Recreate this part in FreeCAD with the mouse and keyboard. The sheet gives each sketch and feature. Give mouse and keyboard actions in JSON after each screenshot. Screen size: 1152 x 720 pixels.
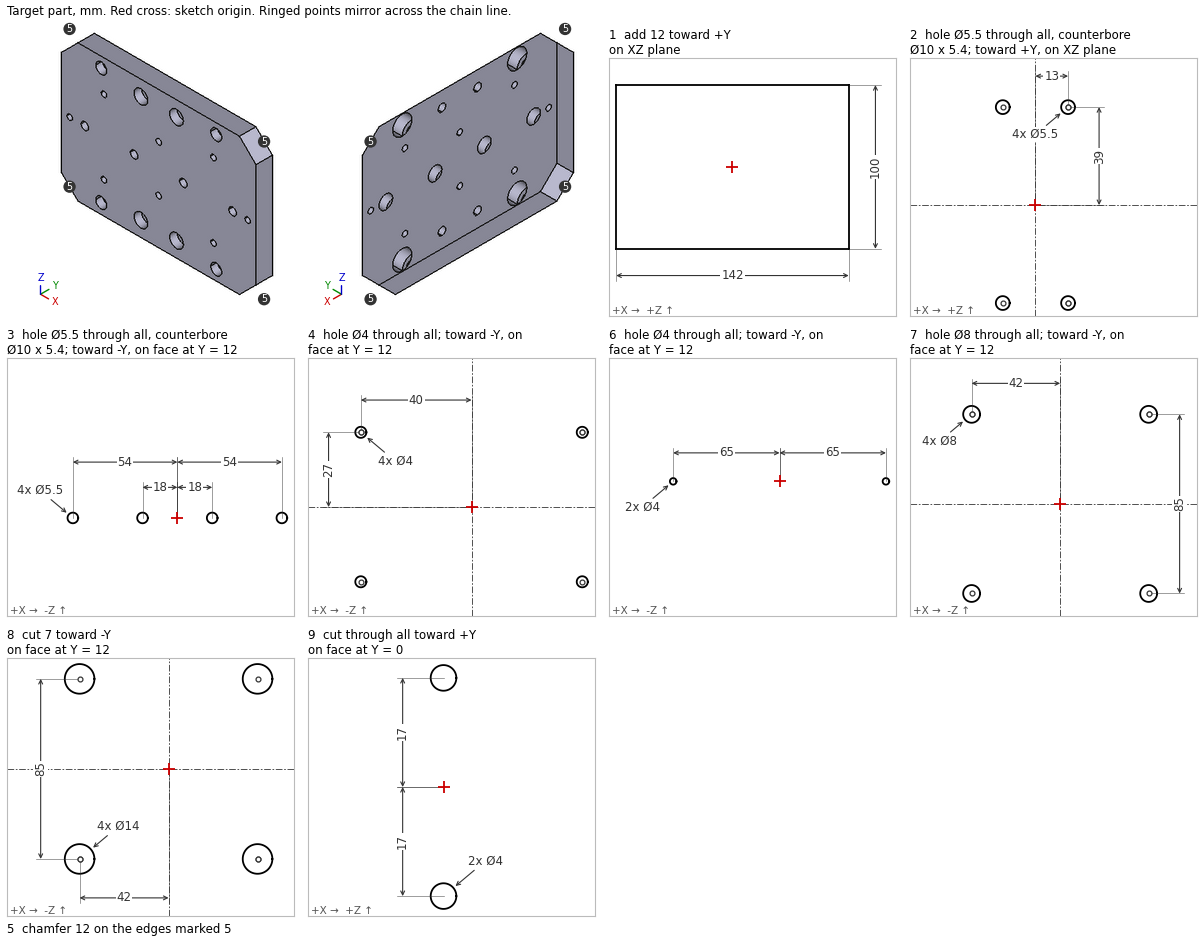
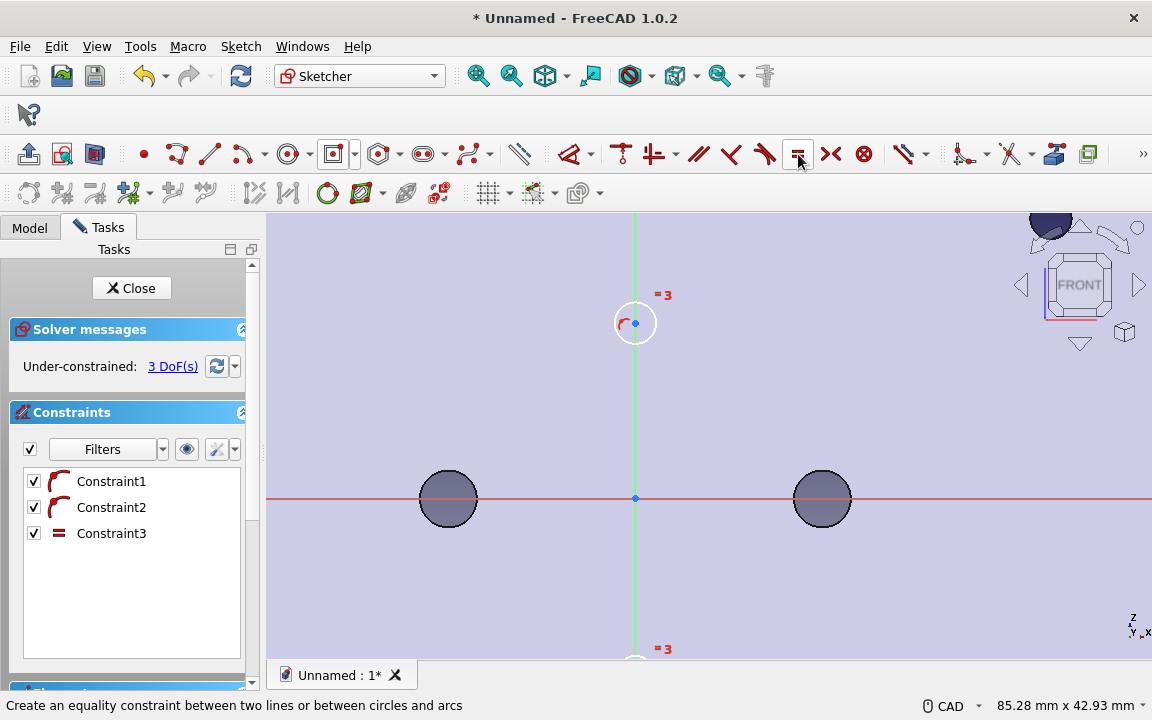
{"action": "left_click", "coordinate": [568, 154]}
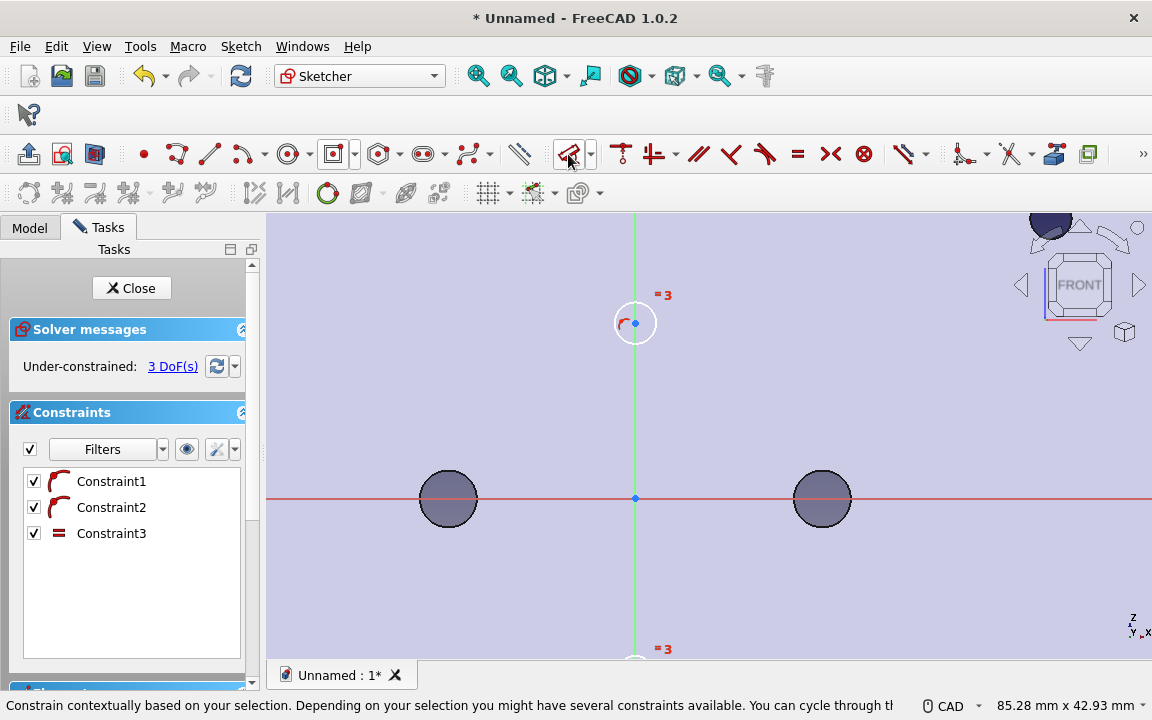
{"action": "scroll", "coordinate": [651, 308], "scroll_direction": "down", "scroll_amount": 2}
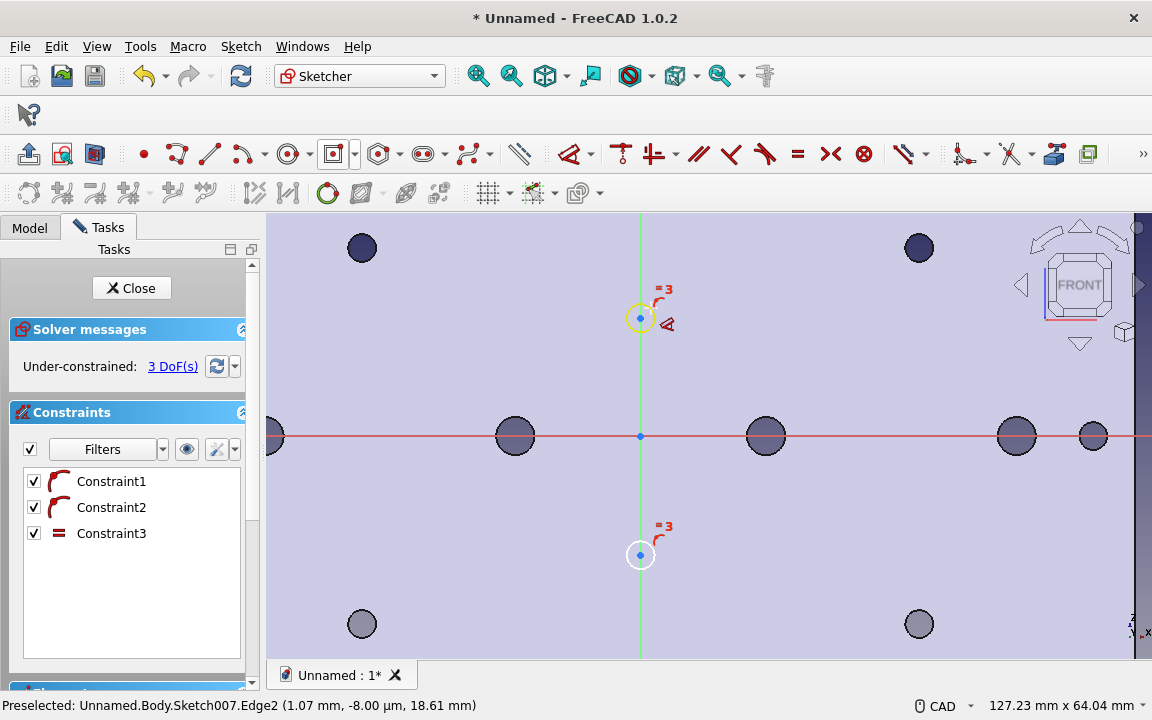
{"action": "scroll", "coordinate": [650, 545], "scroll_direction": "up", "scroll_amount": 2}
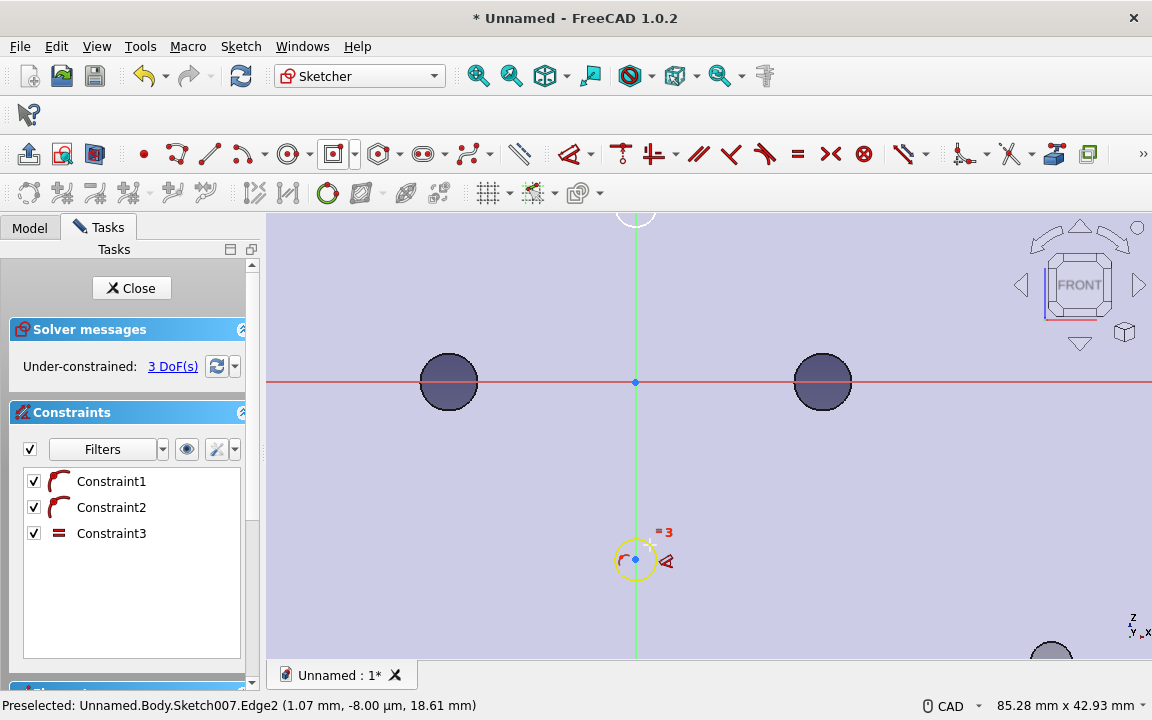
{"action": "left_click", "coordinate": [650, 545]}
{"action": "left_click", "coordinate": [672, 522]}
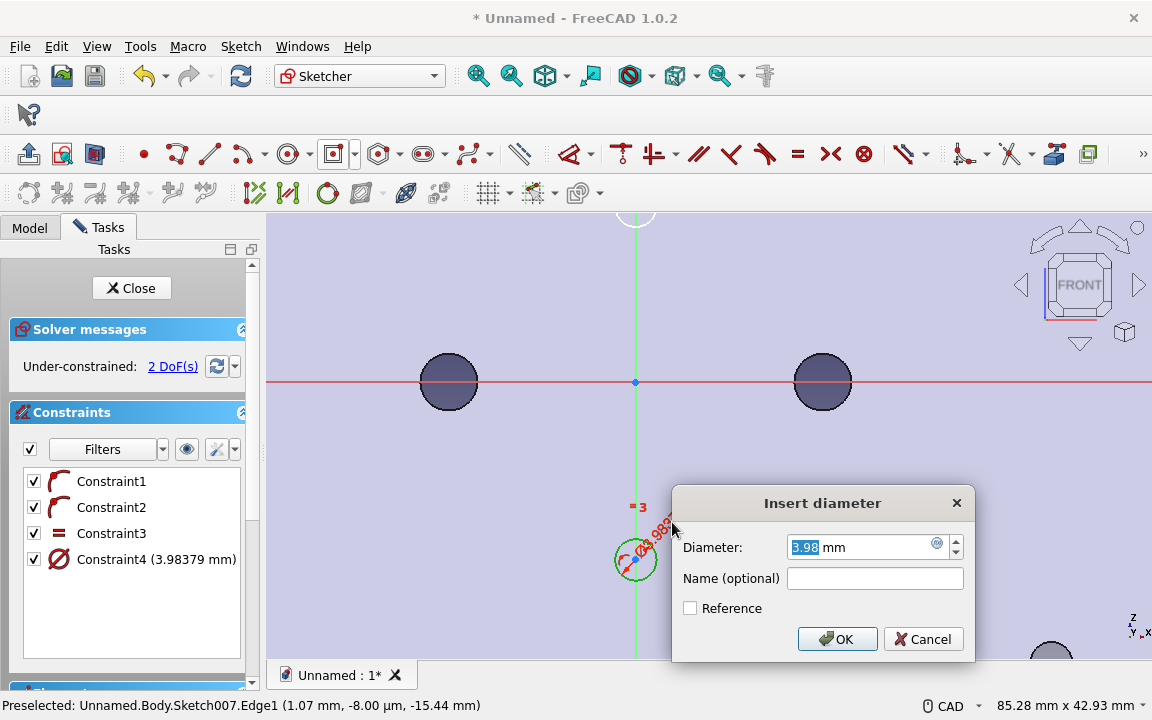
{"action": "type", "text": "4"}
{"action": "key", "text": "Return"}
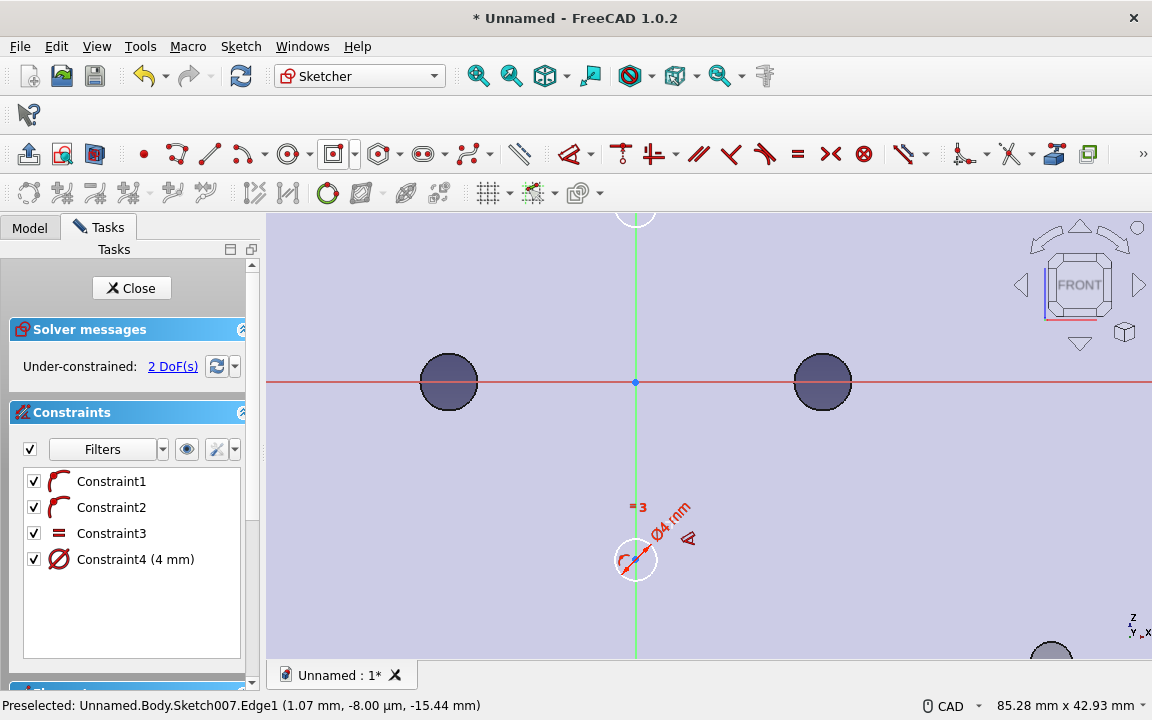
{"action": "left_click", "coordinate": [636, 560]}
{"action": "left_click", "coordinate": [670, 471]}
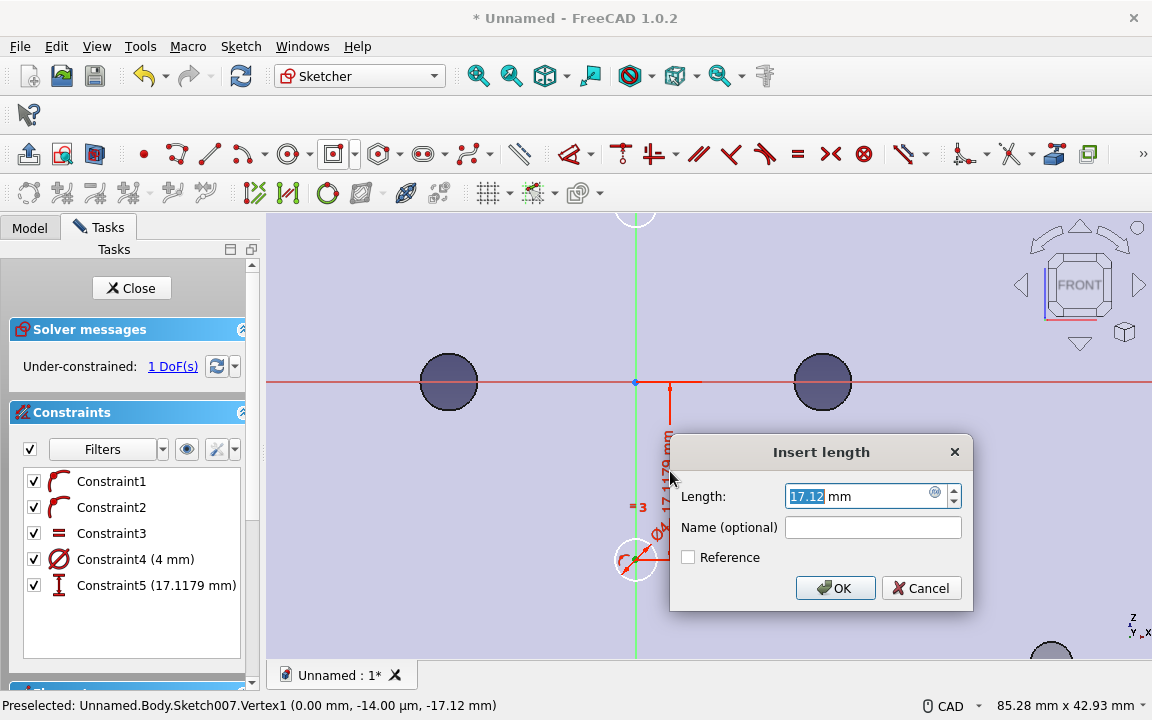
{"action": "type", "text": "17"}
{"action": "key", "text": "Return"}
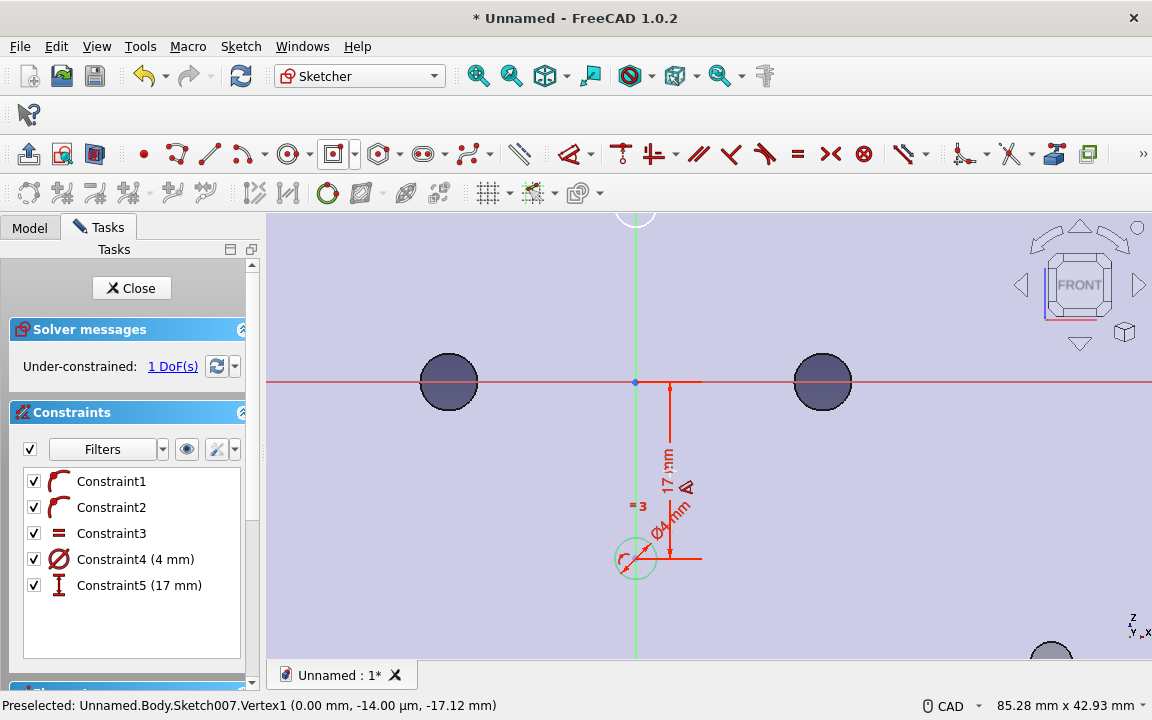
{"action": "scroll", "coordinate": [650, 546], "scroll_direction": "down", "scroll_amount": 2}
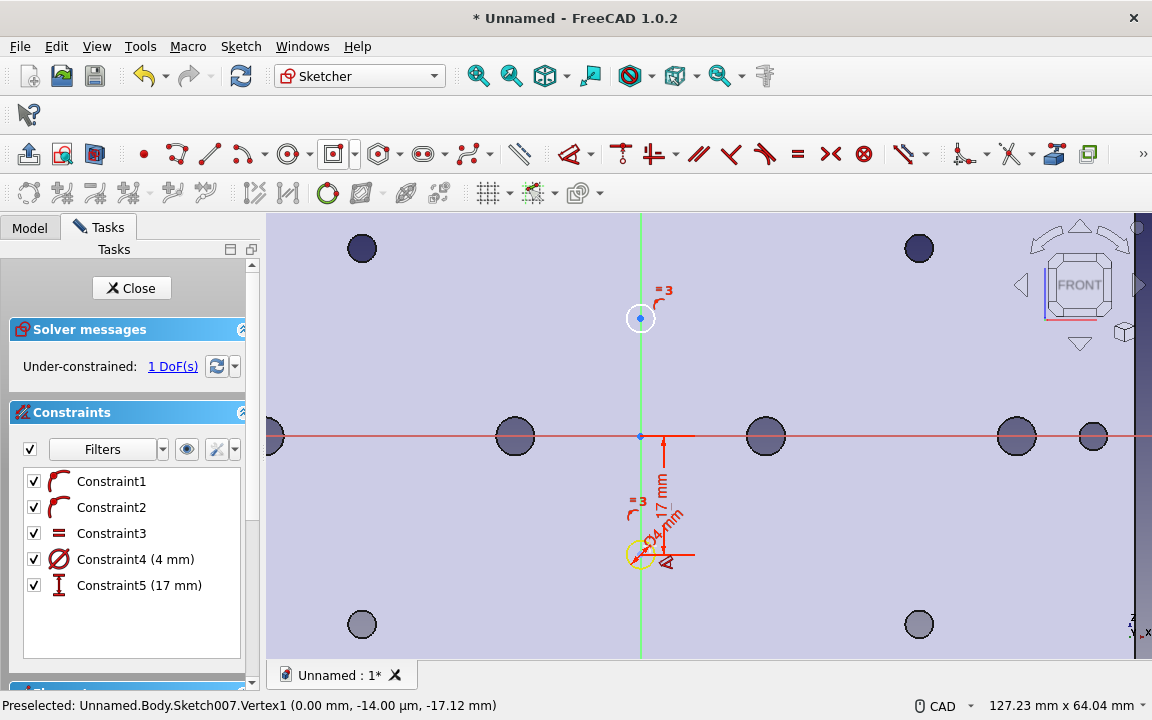
{"action": "left_click", "coordinate": [641, 319]}
{"action": "left_click", "coordinate": [675, 377]}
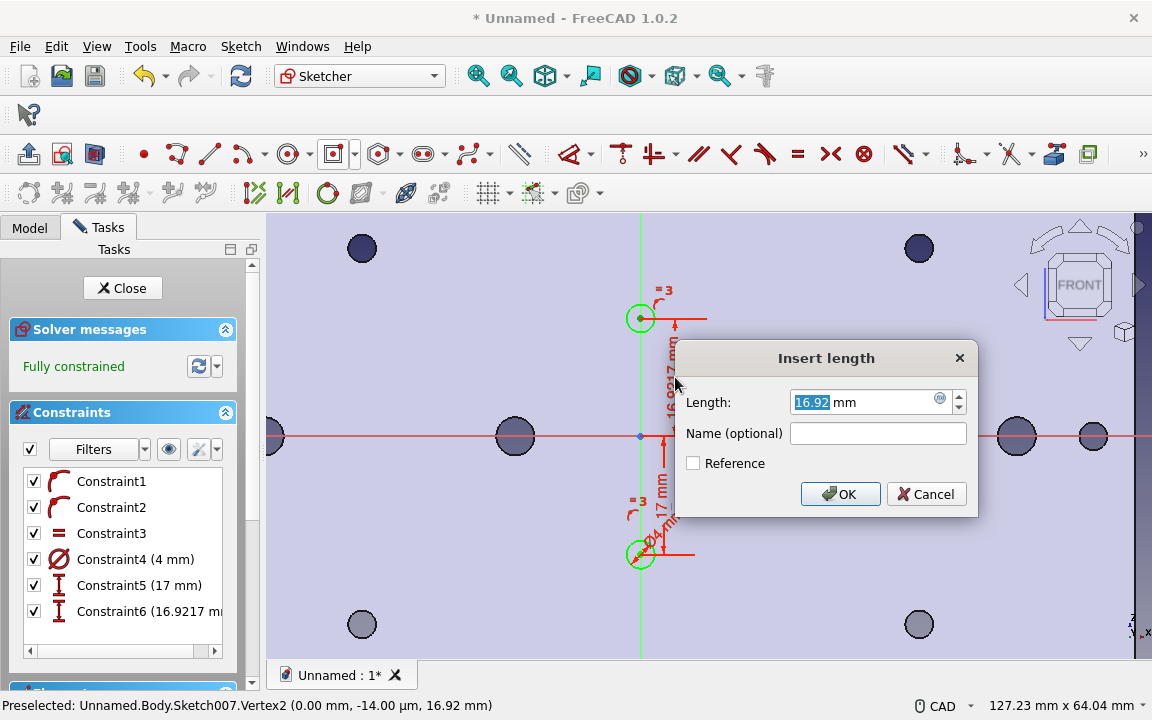
{"action": "type", "text": "17"}
{"action": "key", "text": "Return"}
{"action": "key", "text": "Escape"}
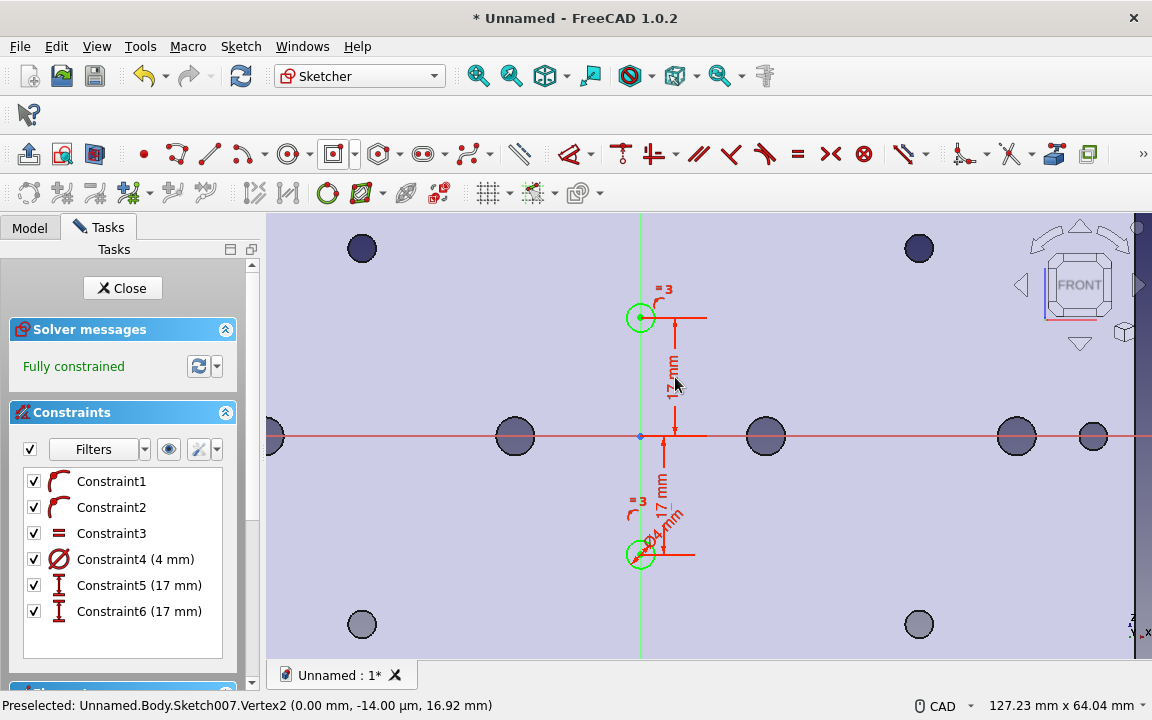
{"action": "left_click", "coordinate": [123, 288]}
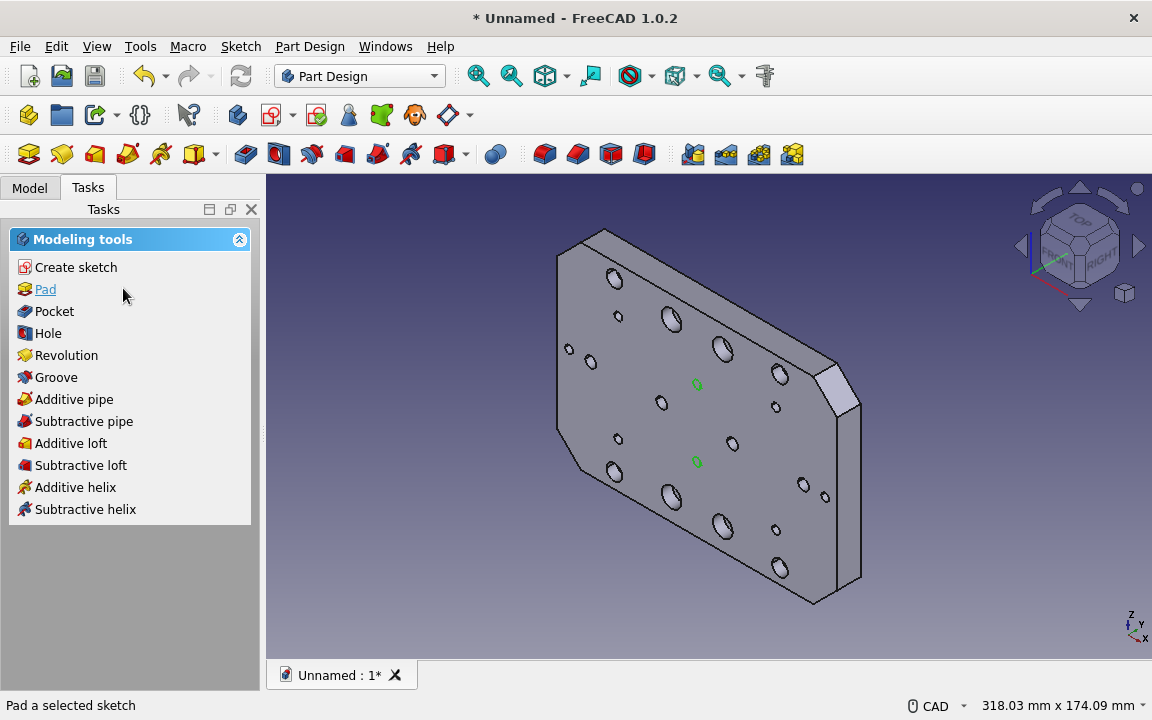
{"action": "left_click", "coordinate": [246, 154]}